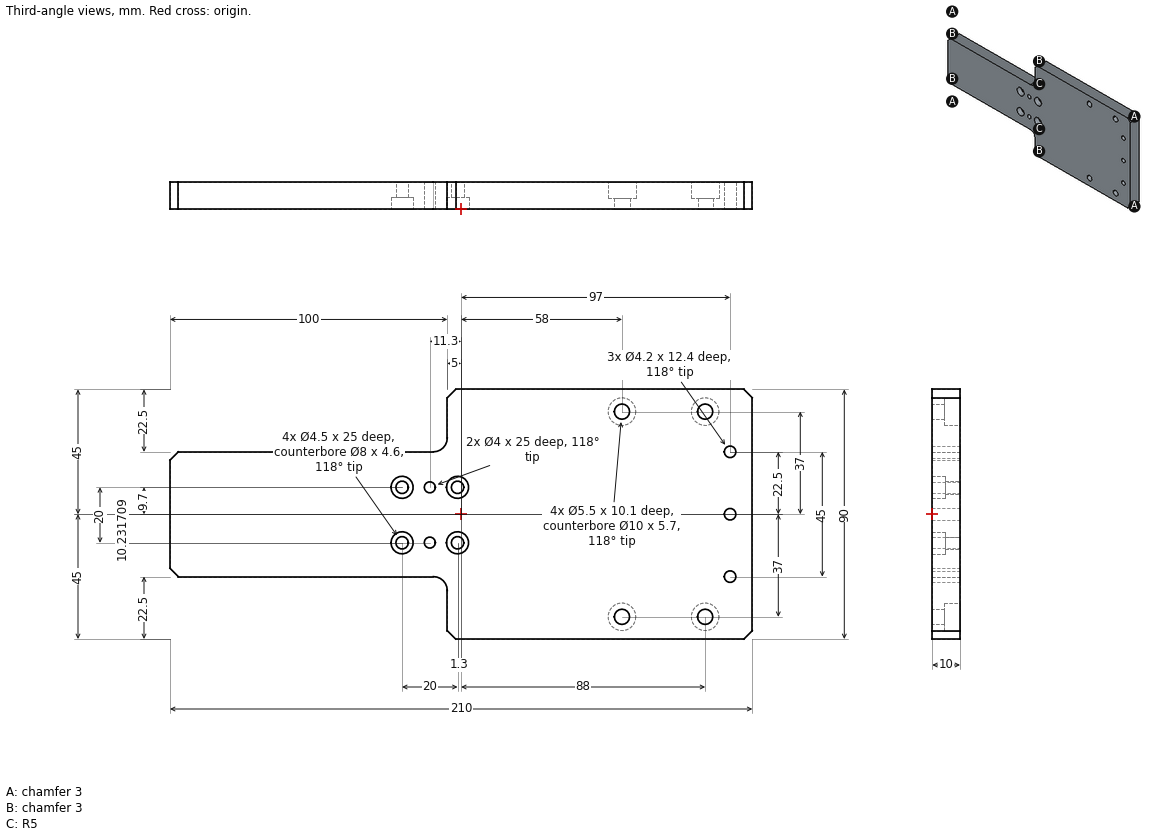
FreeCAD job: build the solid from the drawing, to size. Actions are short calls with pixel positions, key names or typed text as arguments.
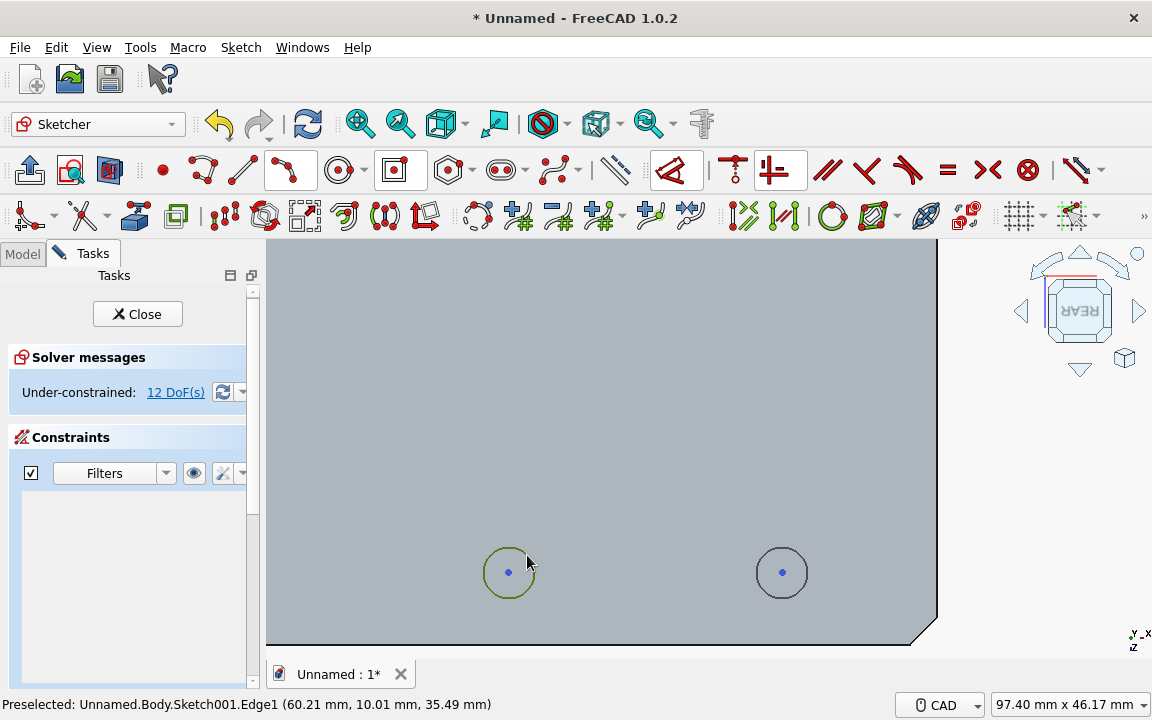
scroll(784, 573, down, 5)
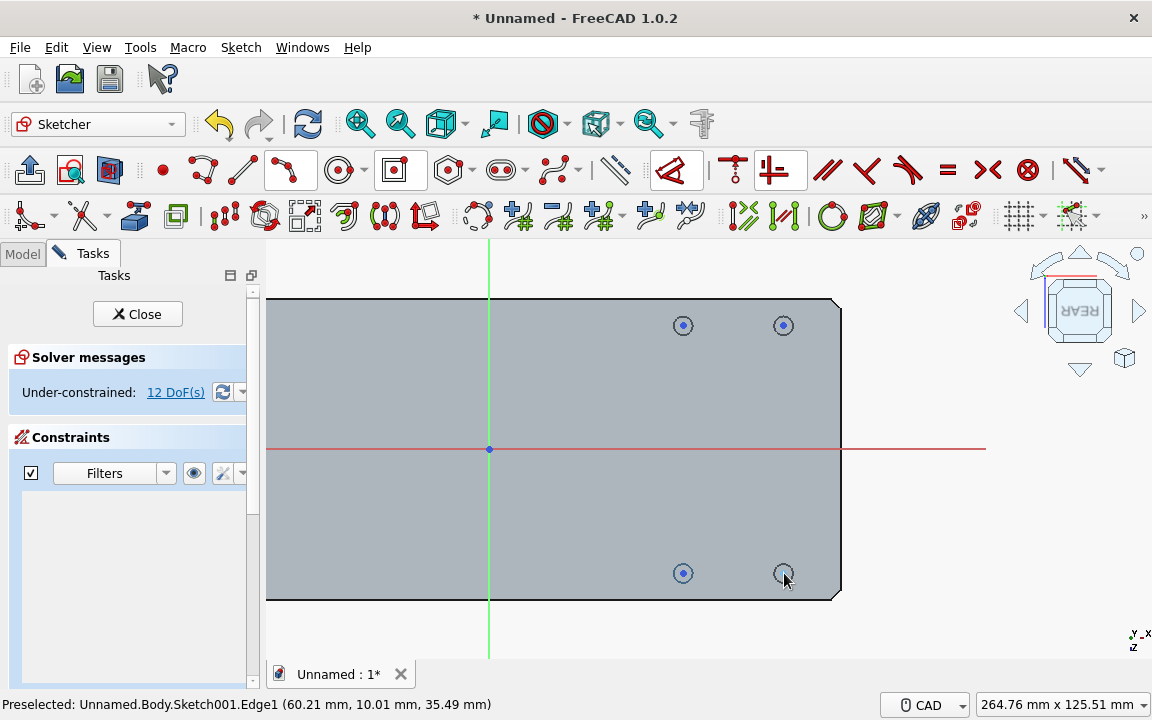
scroll(690, 319, up, 2)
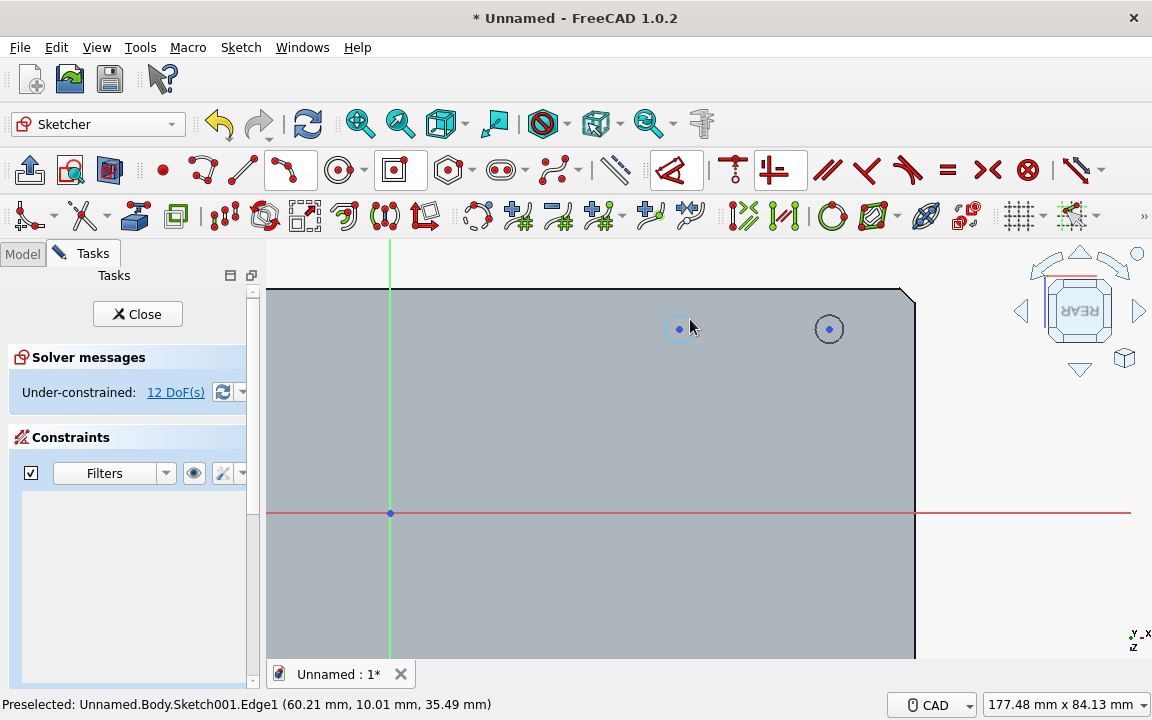
click(689, 319)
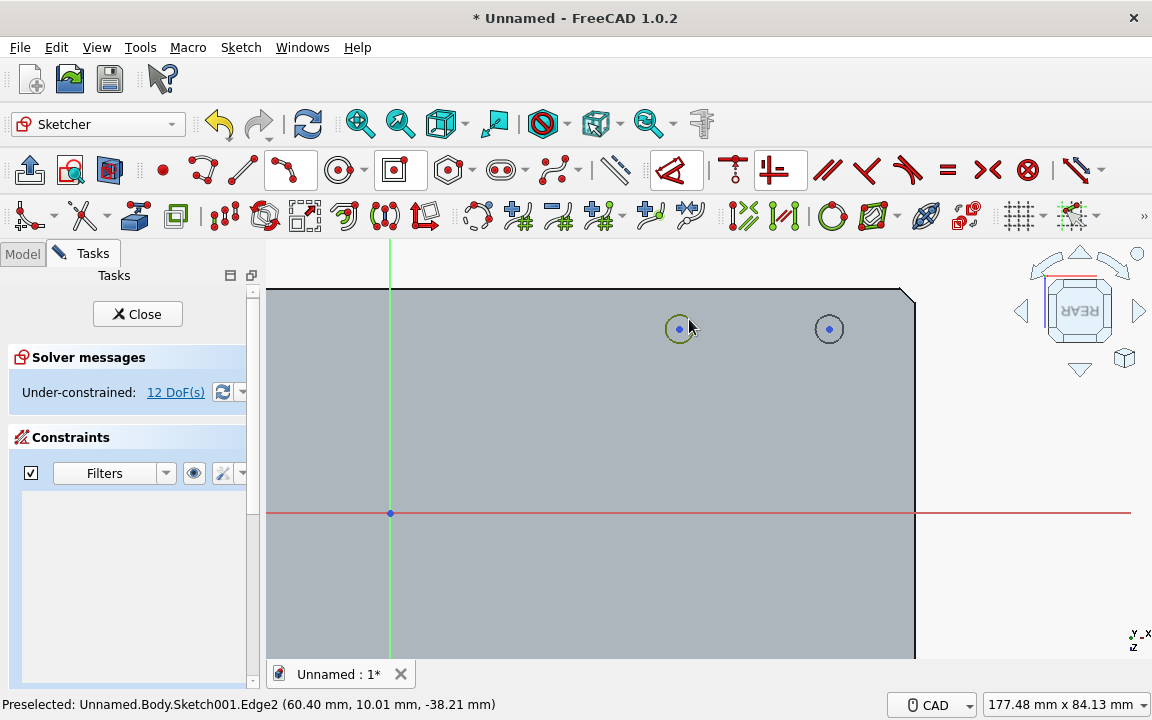
click(839, 319)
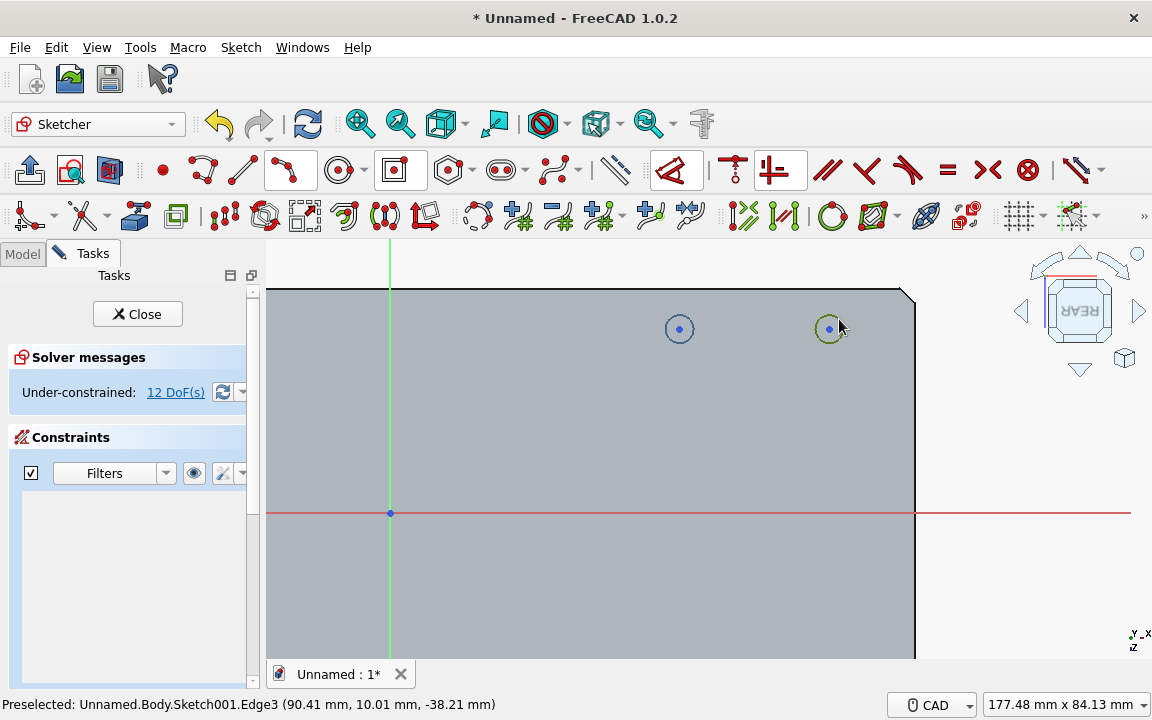
scroll(689, 319, down, 2)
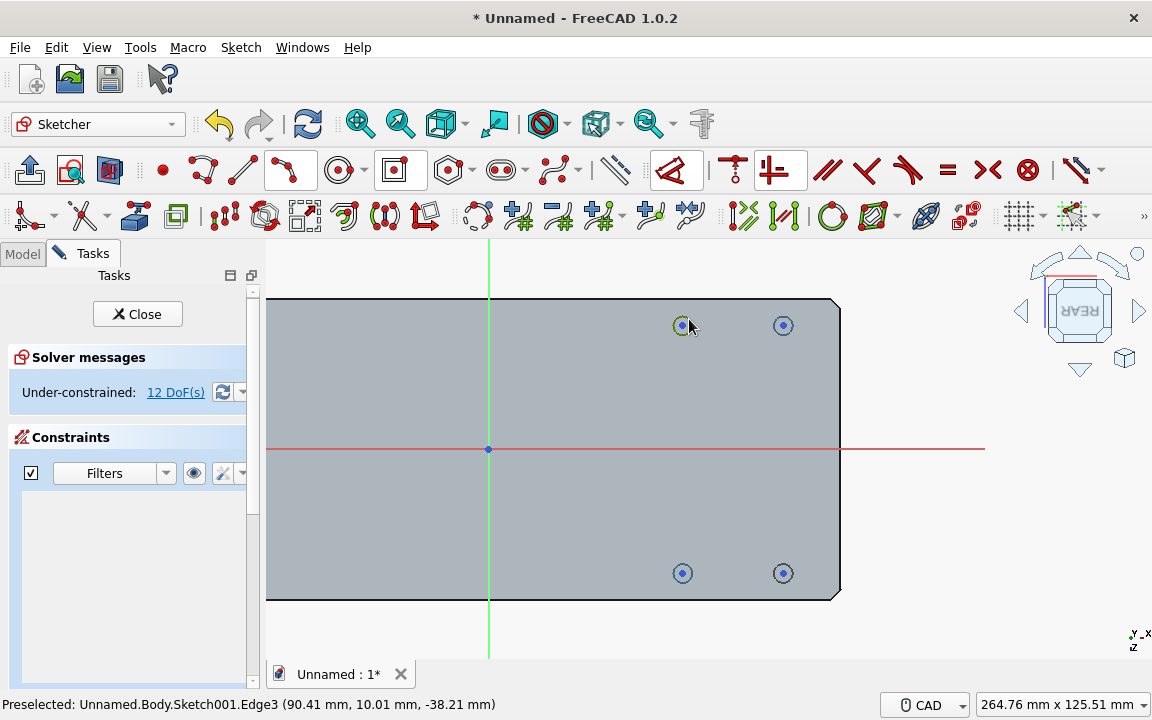
scroll(790, 567, up, 2)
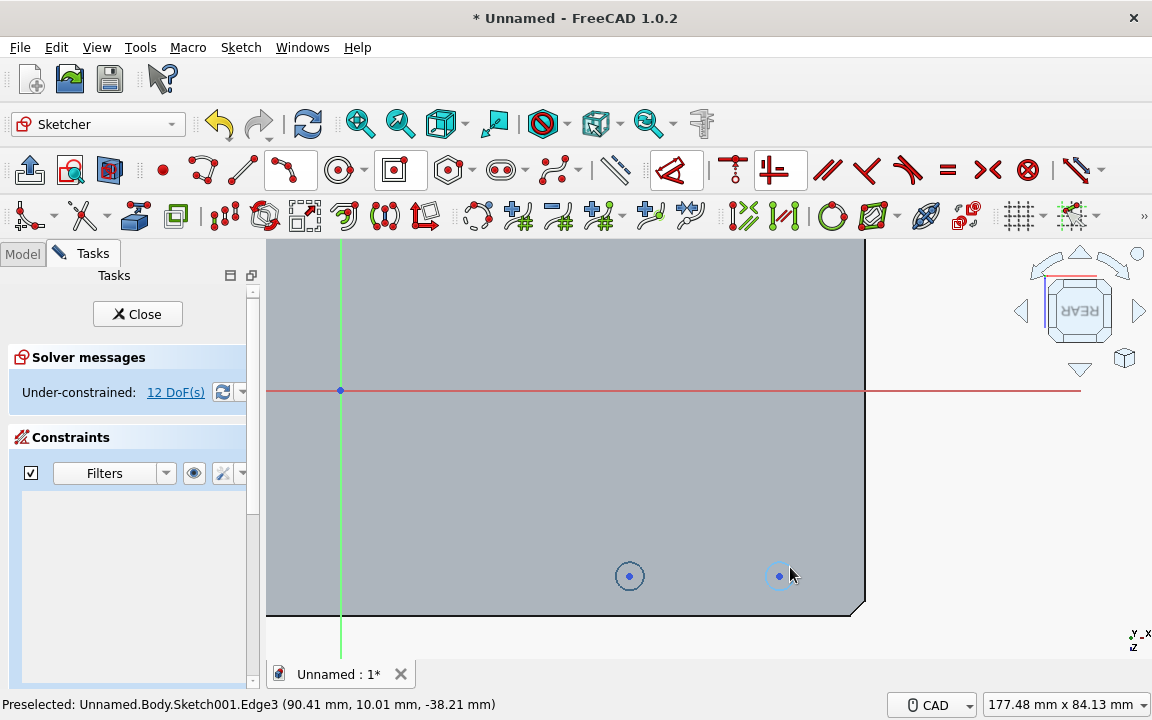
click(790, 566)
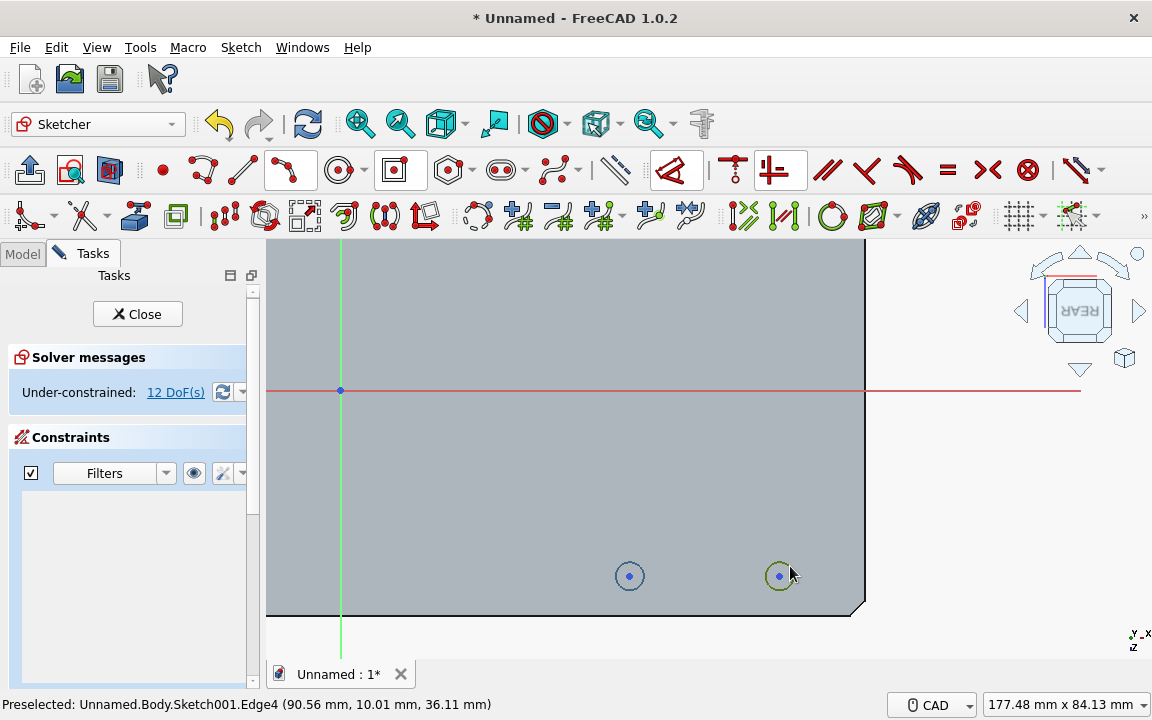
click(948, 170)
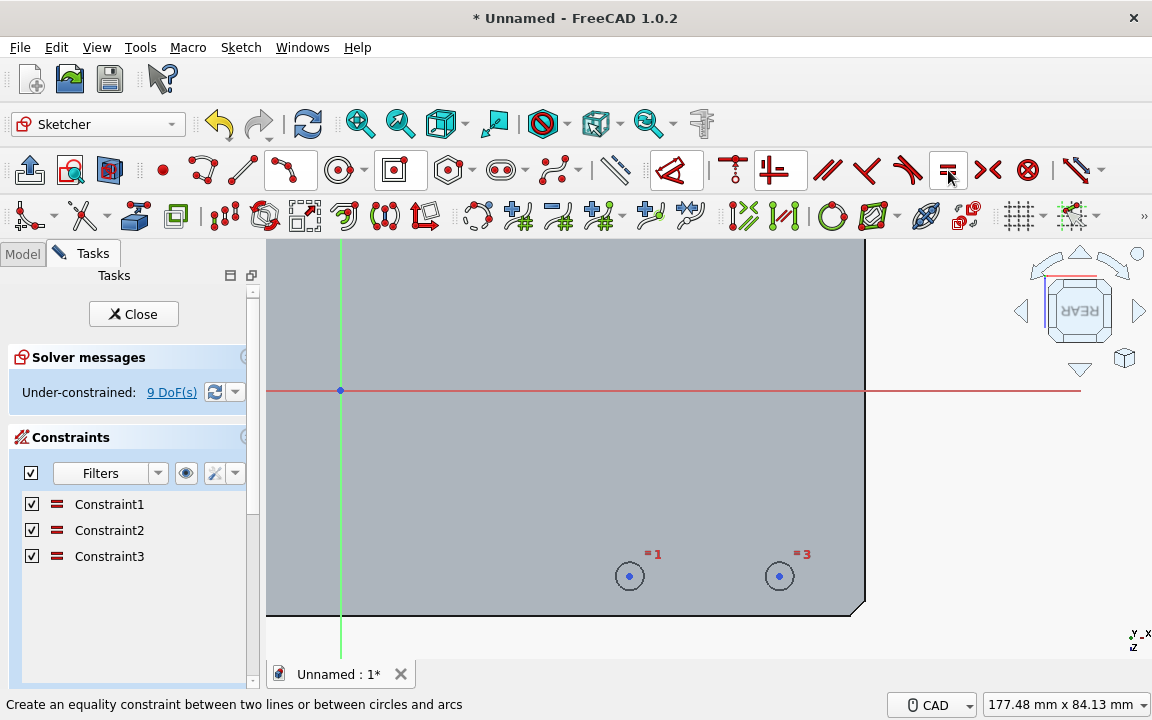
click(630, 576)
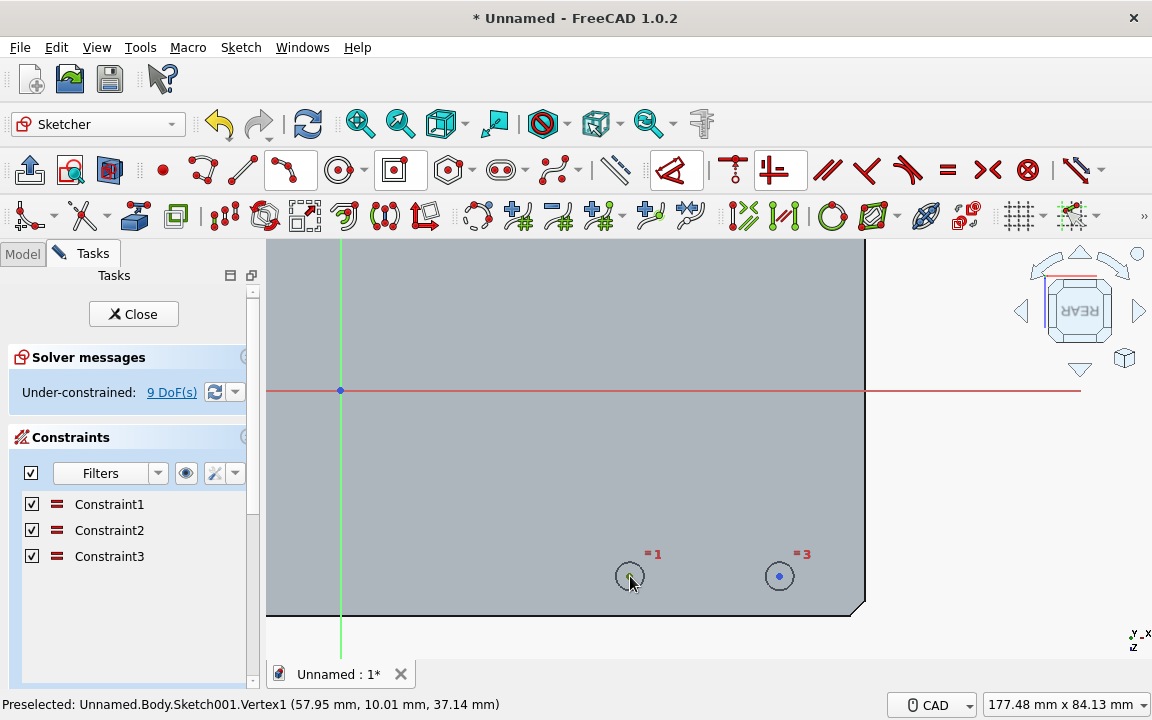
scroll(790, 567, down, 2)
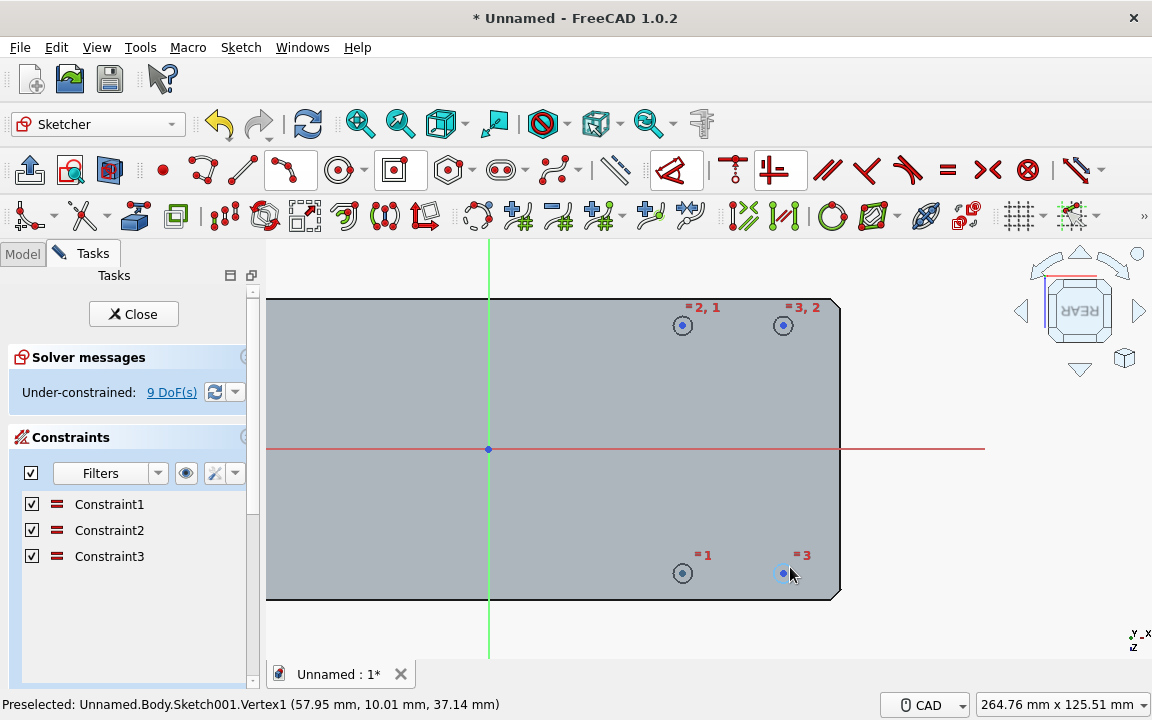
click(683, 326)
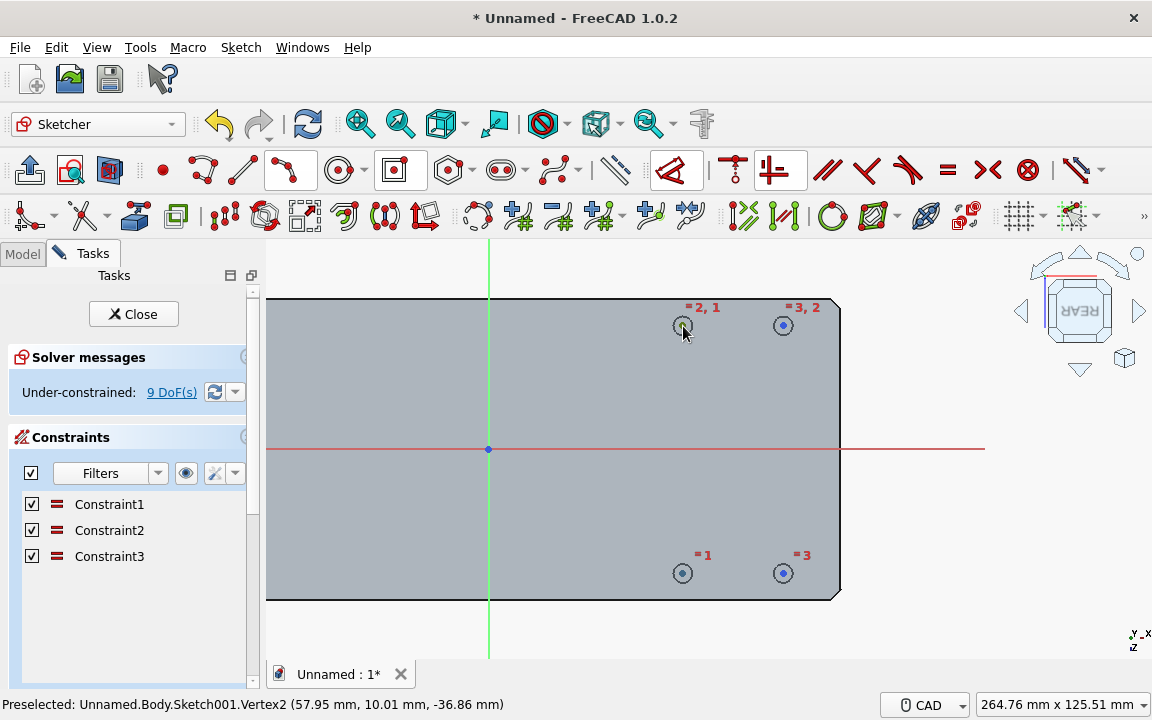
click(802, 170)